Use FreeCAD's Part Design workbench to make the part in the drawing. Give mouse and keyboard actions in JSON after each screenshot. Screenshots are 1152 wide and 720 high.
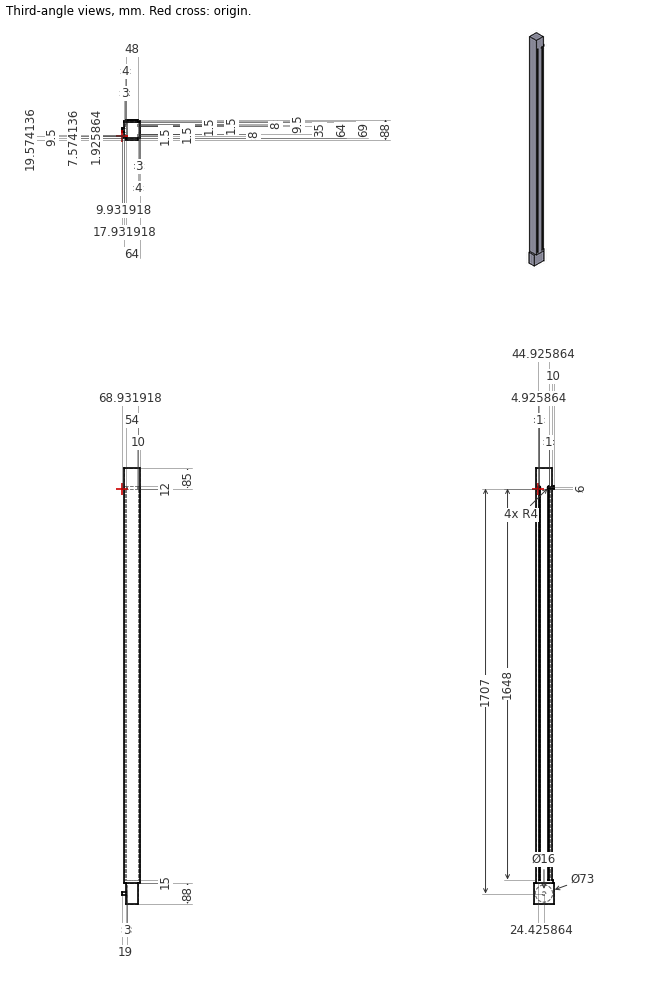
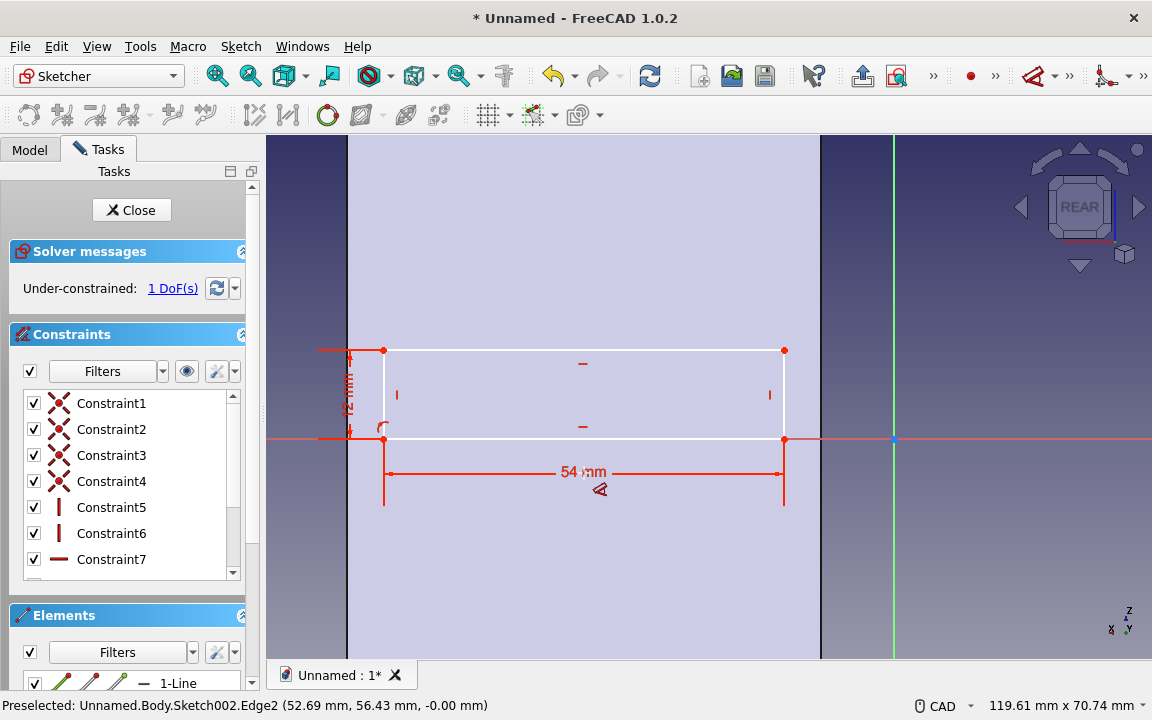
{"action": "left_click", "coordinate": [384, 350]}
{"action": "left_click", "coordinate": [757, 473]}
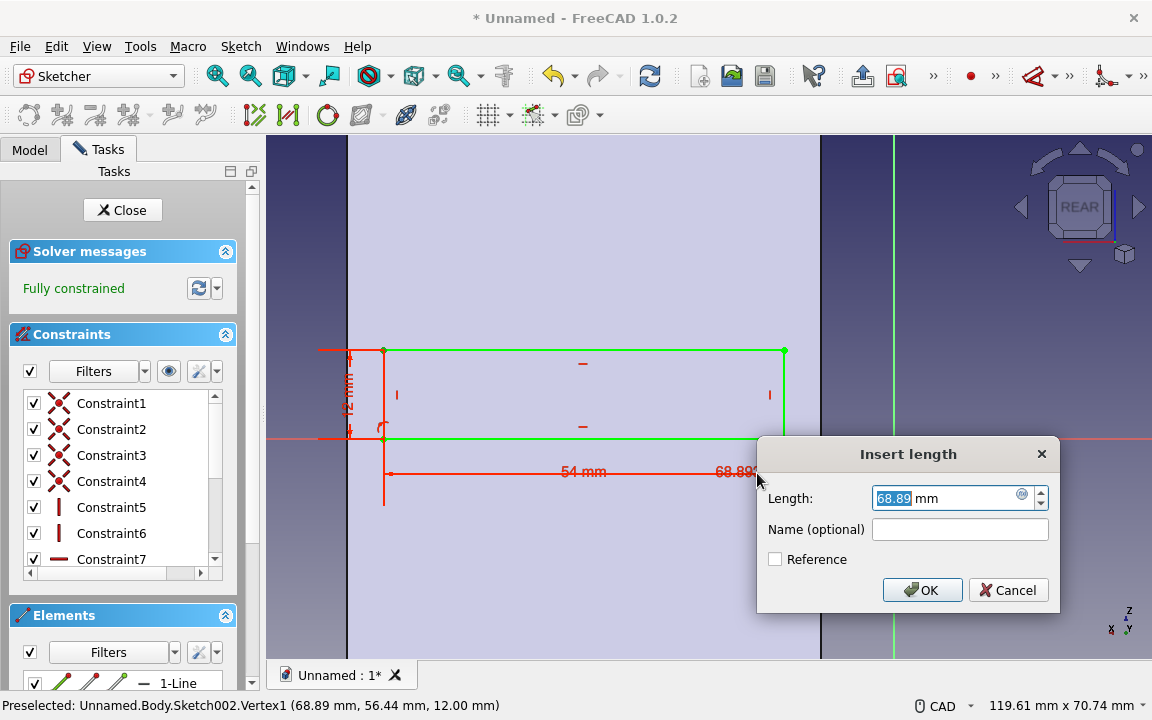
{"action": "type", "text": "68.931918"}
{"action": "key", "text": "Return"}
{"action": "key", "text": "Escape"}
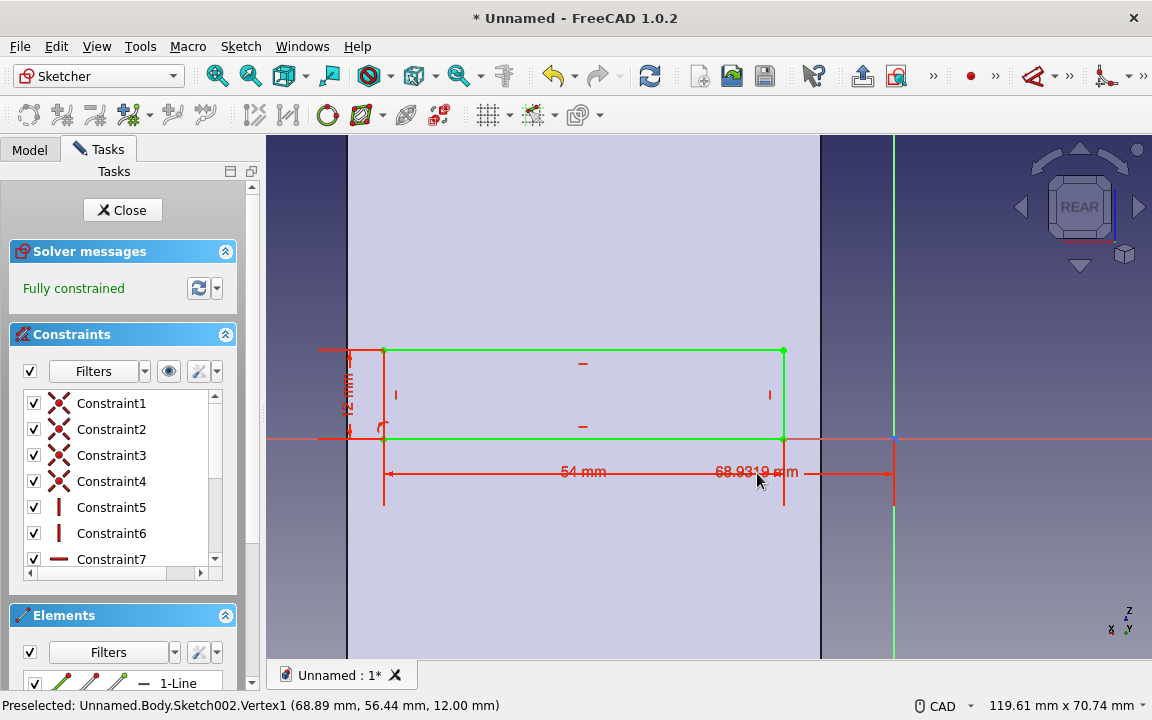
{"action": "left_click", "coordinate": [123, 210]}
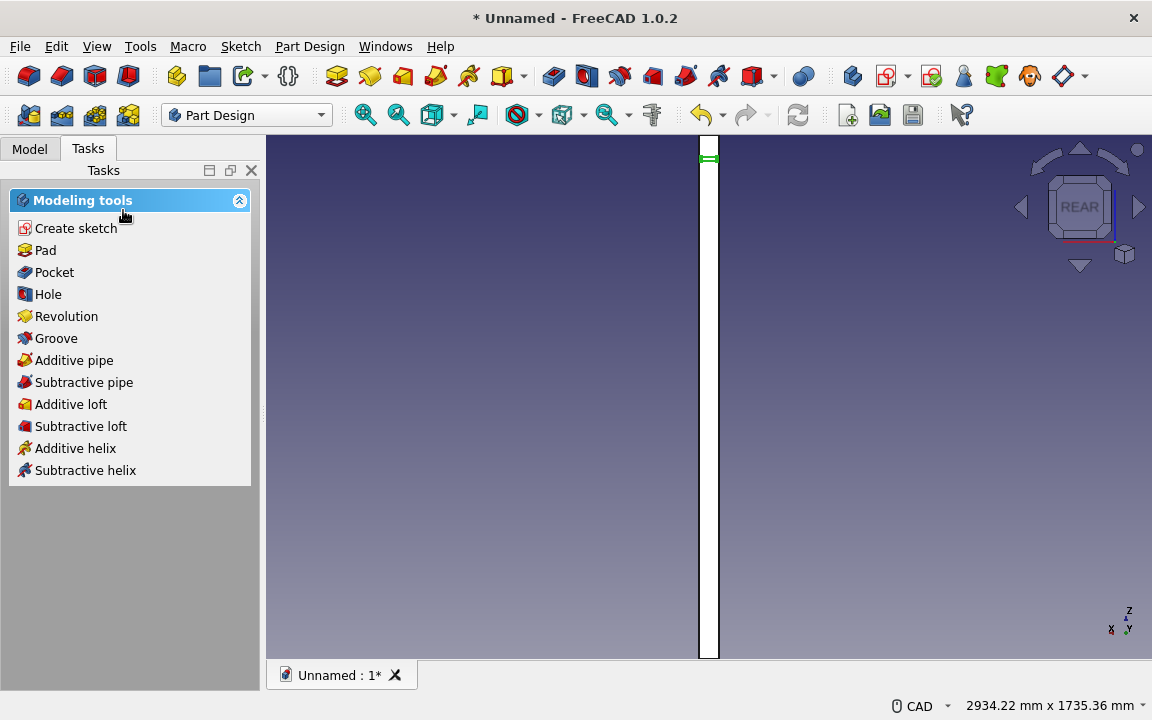
{"action": "left_click", "coordinate": [337, 76]}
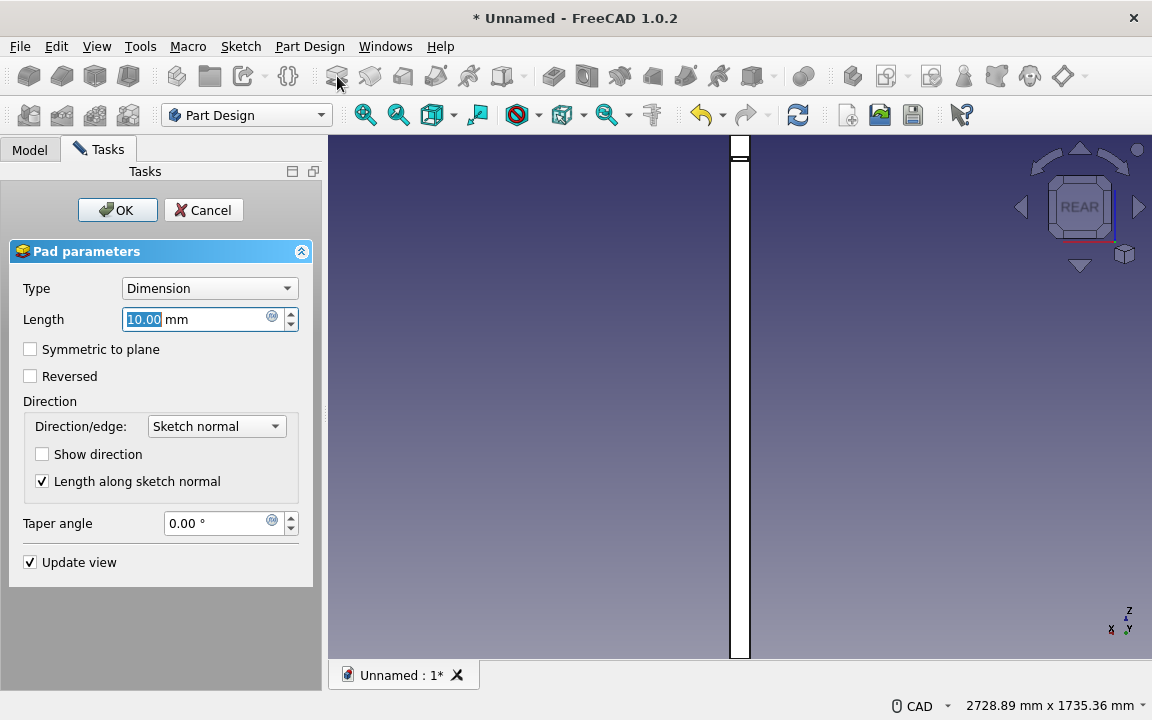
{"action": "type", "text": "10"}
{"action": "key", "text": "Tab"}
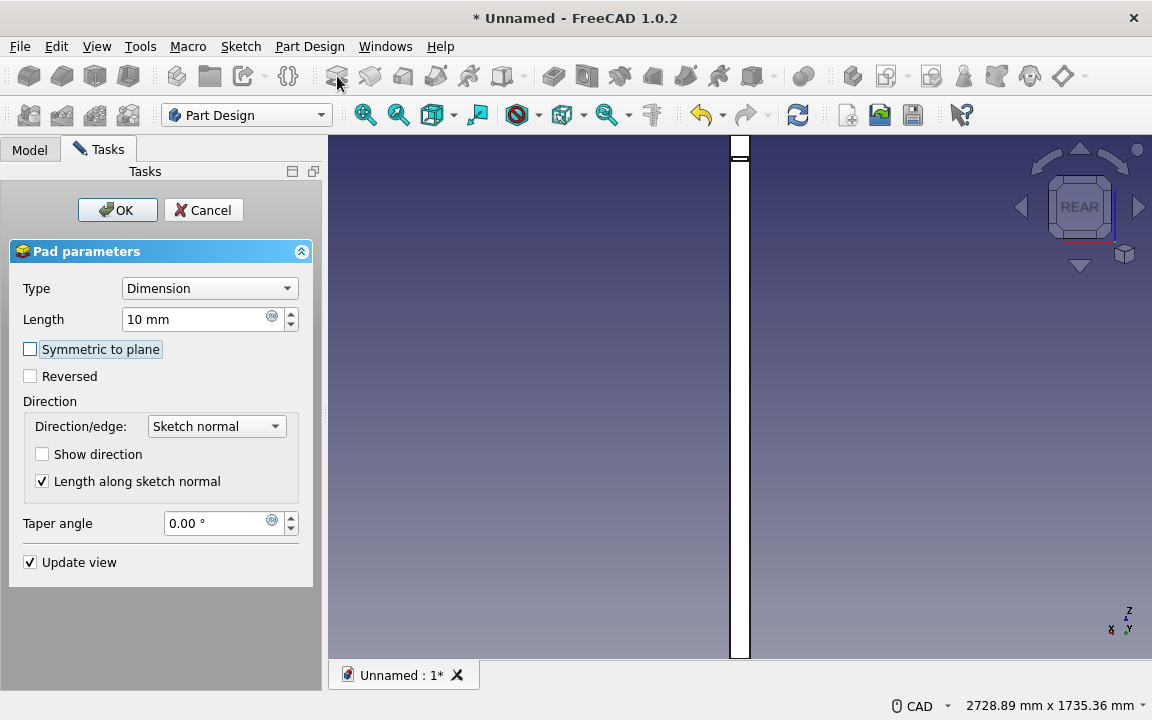
{"action": "left_click", "coordinate": [118, 210]}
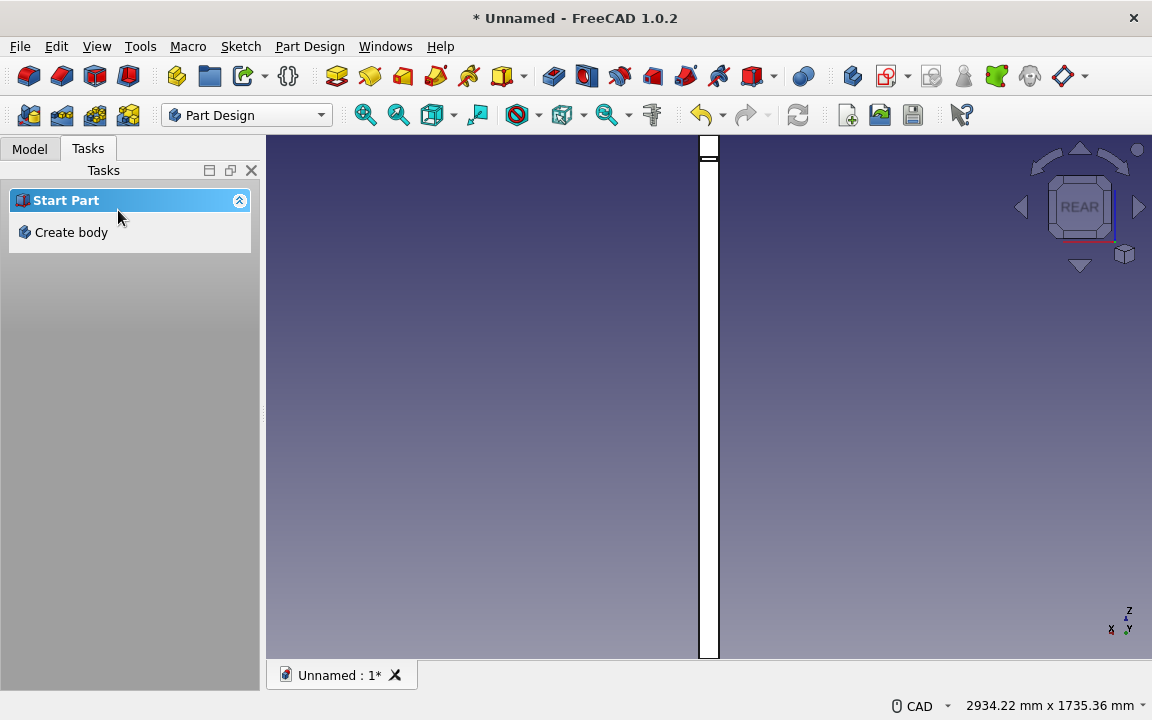
{"action": "left_click", "coordinate": [366, 116]}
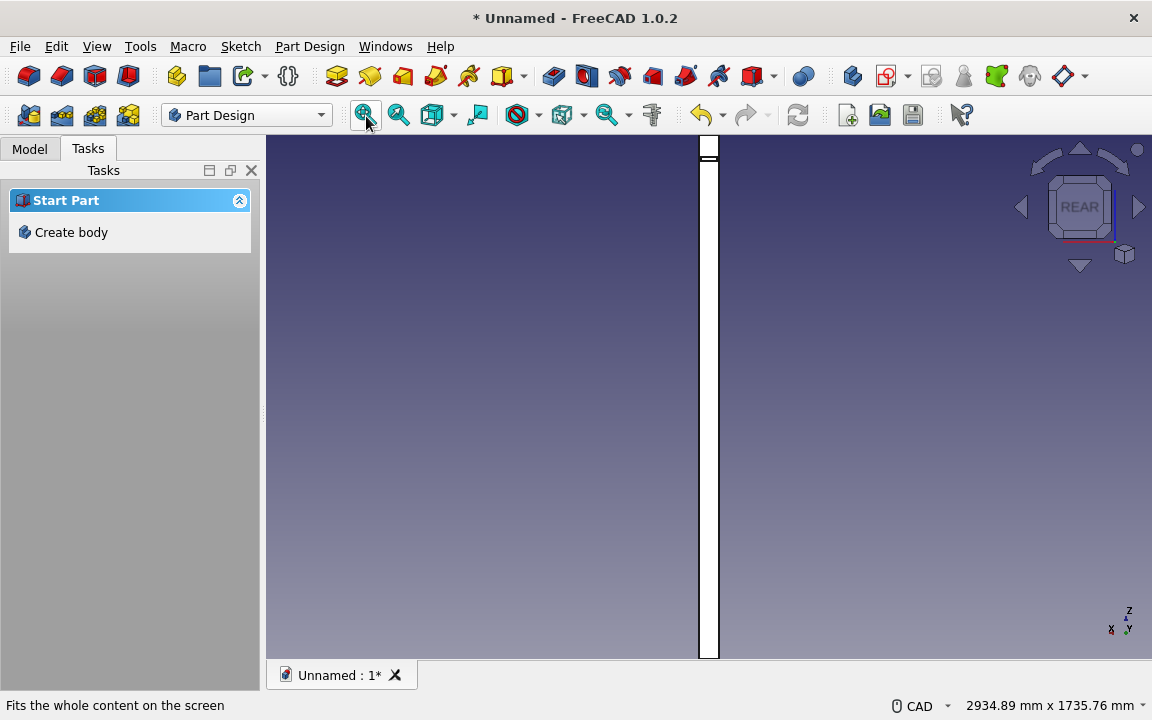
{"action": "key", "text": "0"}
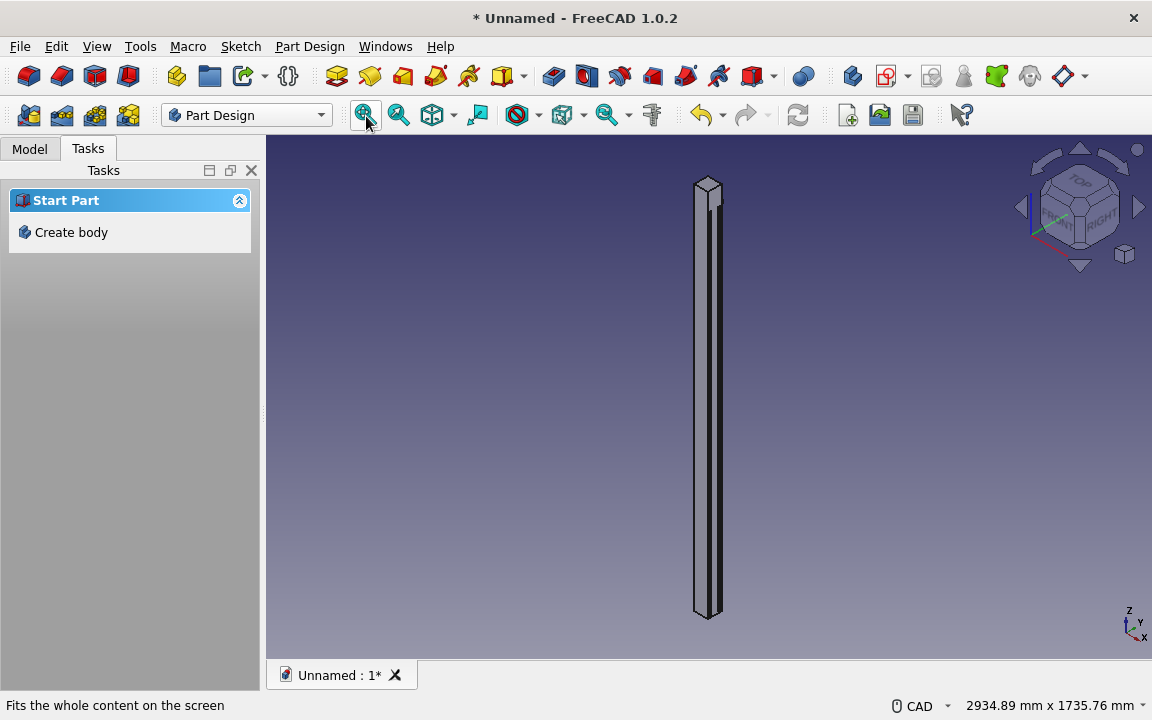
{"action": "scroll", "coordinate": [715, 217], "scroll_direction": "up", "scroll_amount": 5}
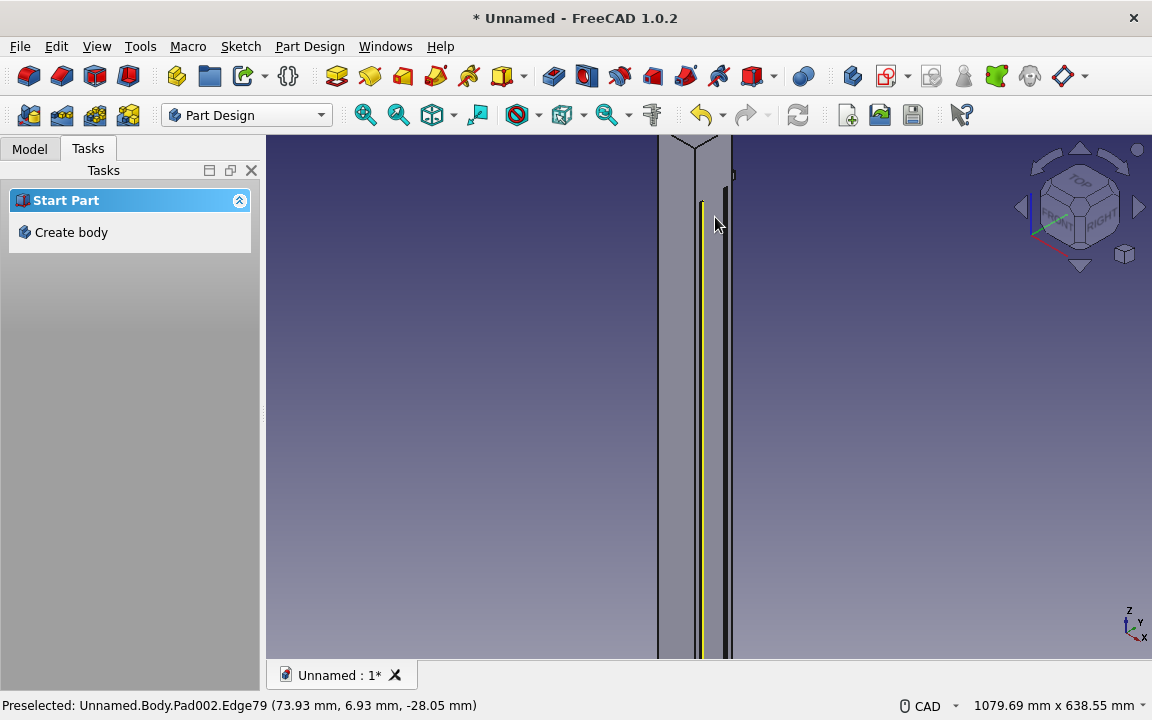
{"action": "left_click", "coordinate": [713, 220]}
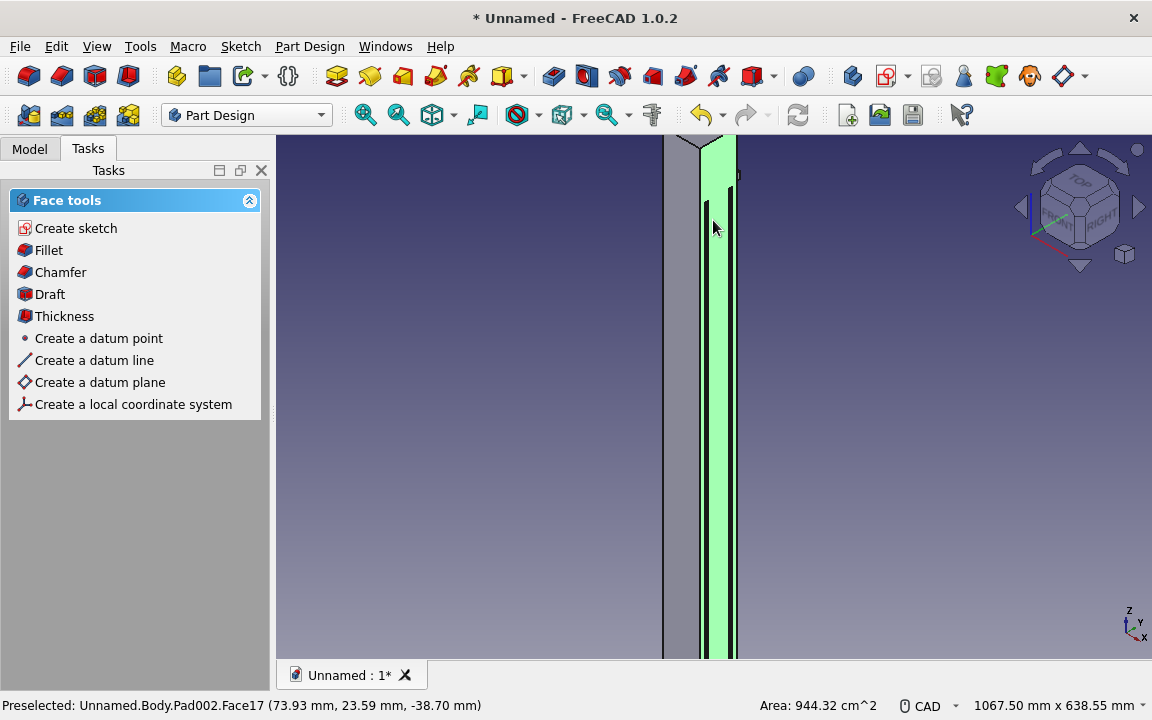
{"action": "left_click", "coordinate": [886, 76]}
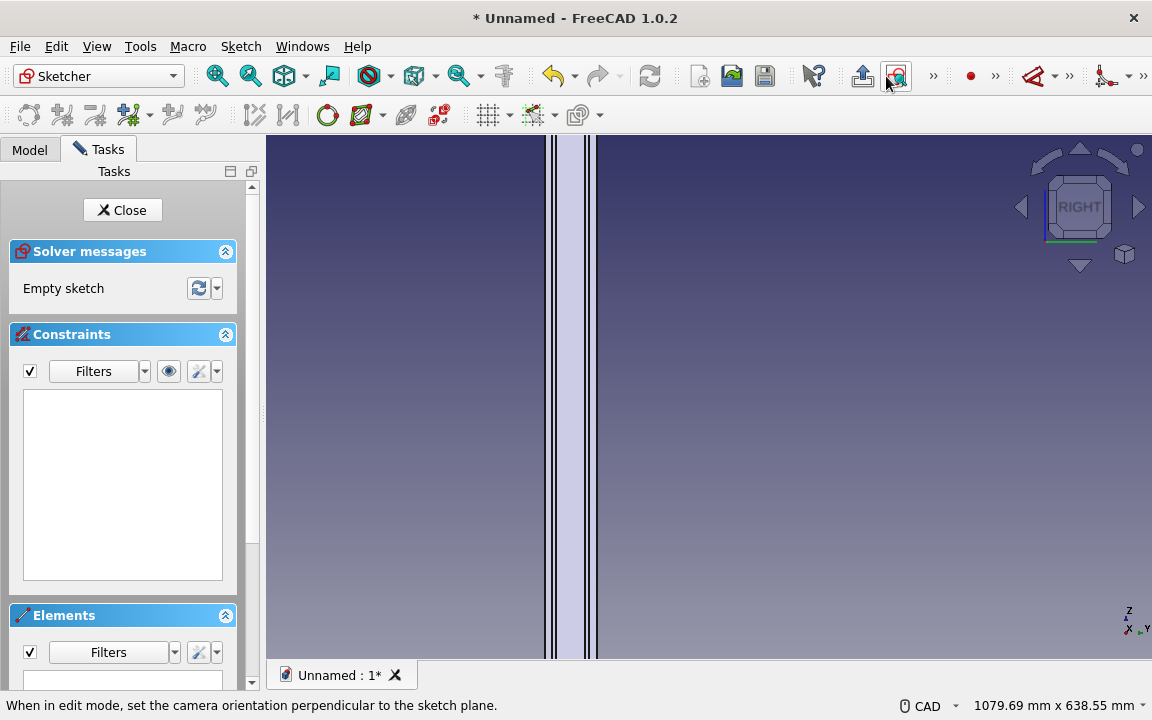
{"action": "scroll", "coordinate": [640, 397], "scroll_direction": "down", "scroll_amount": 5}